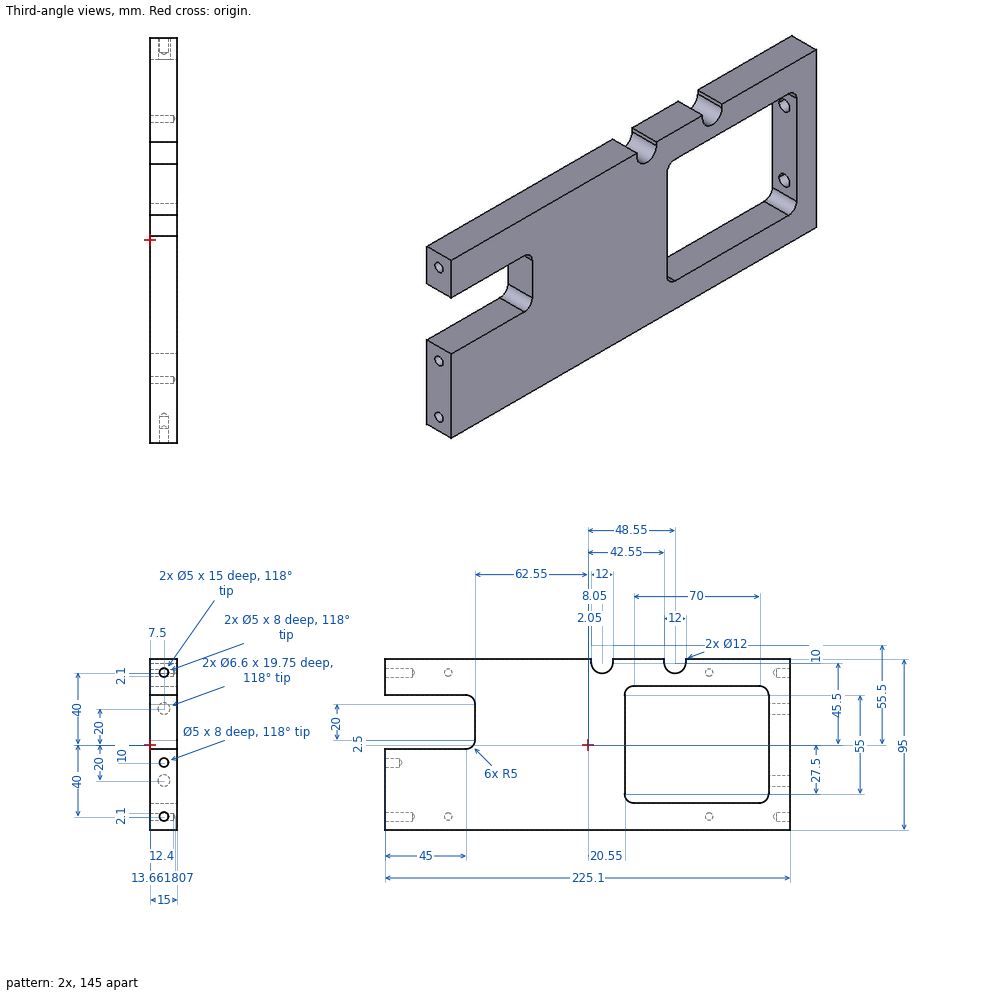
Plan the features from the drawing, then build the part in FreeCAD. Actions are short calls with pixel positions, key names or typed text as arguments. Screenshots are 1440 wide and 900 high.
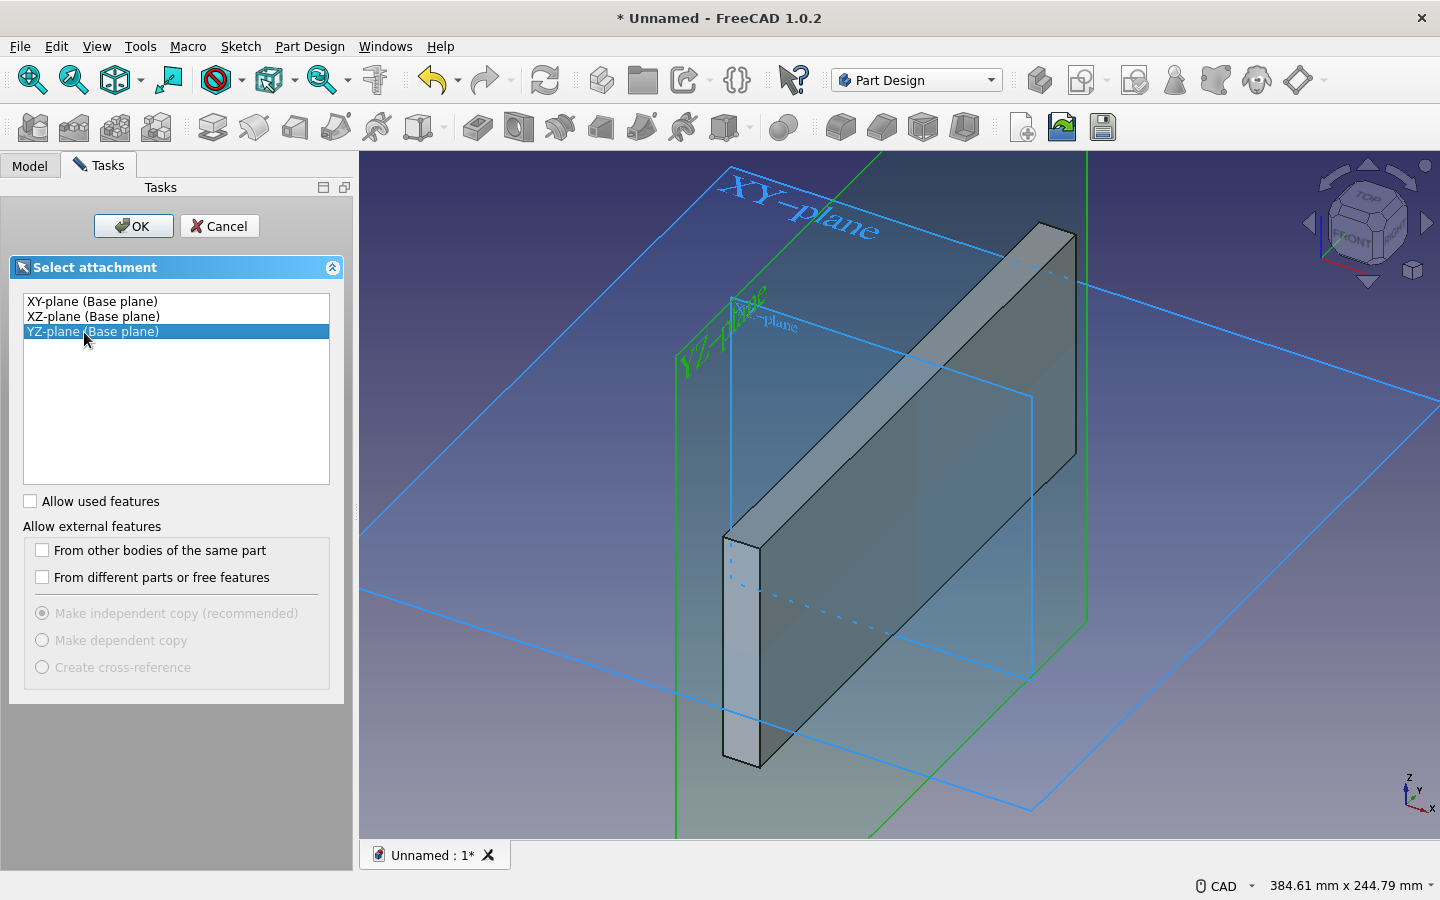
click(134, 226)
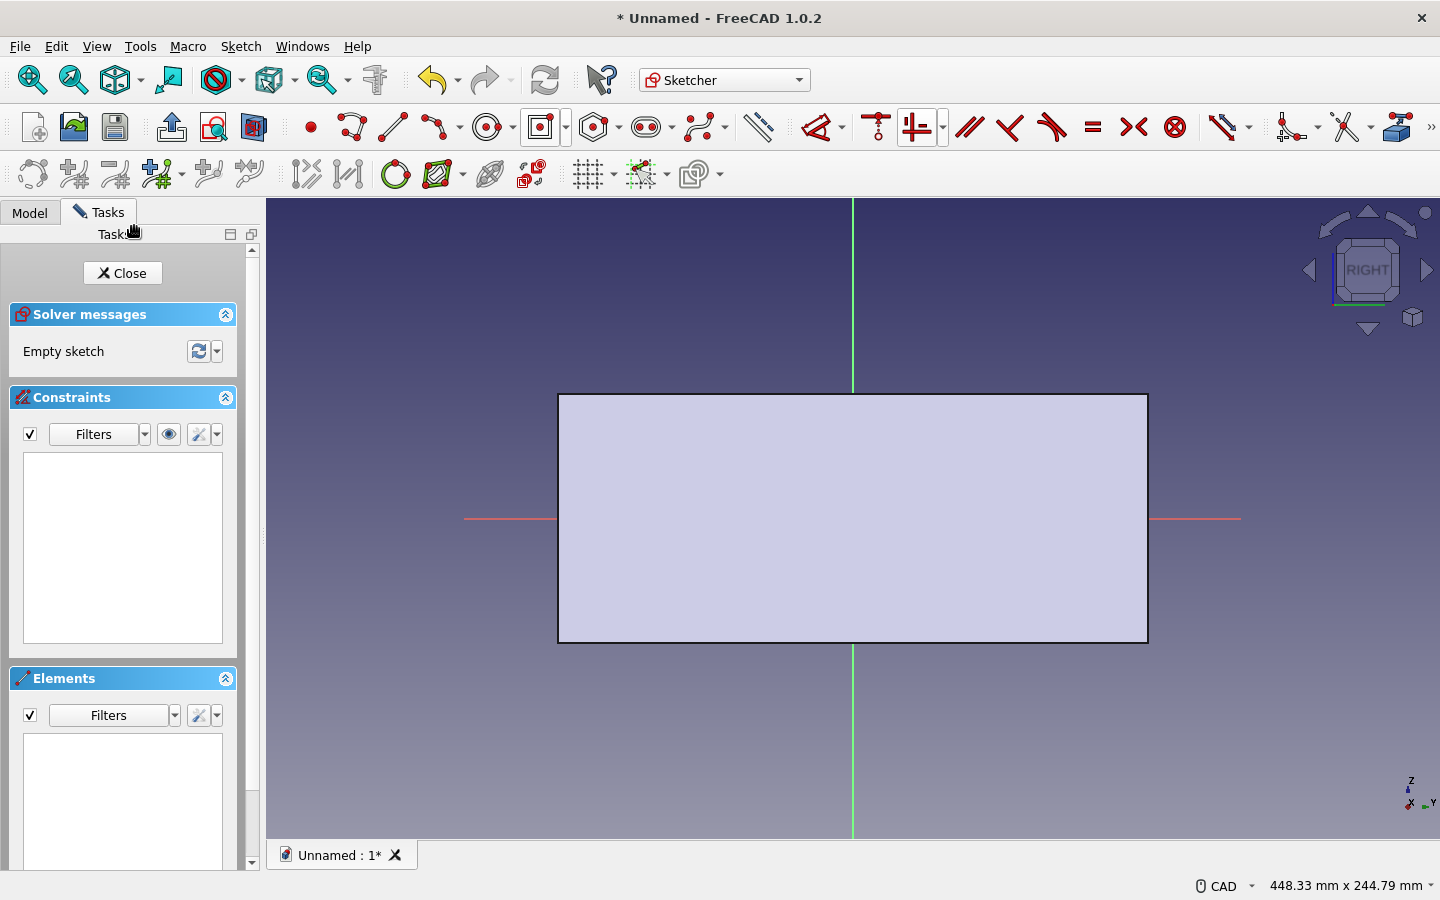
click(254, 128)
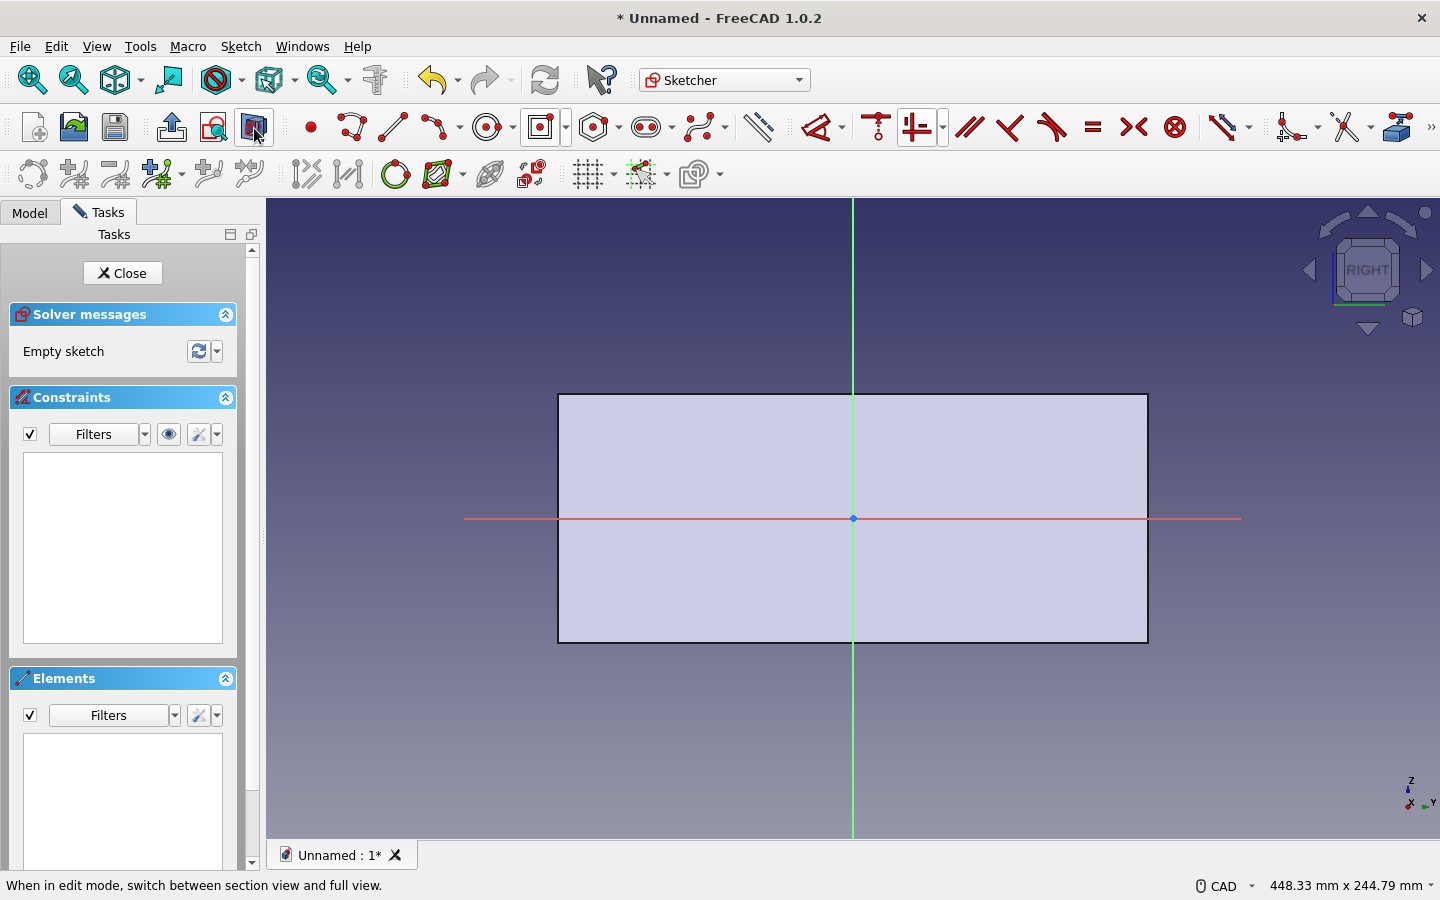
click(393, 128)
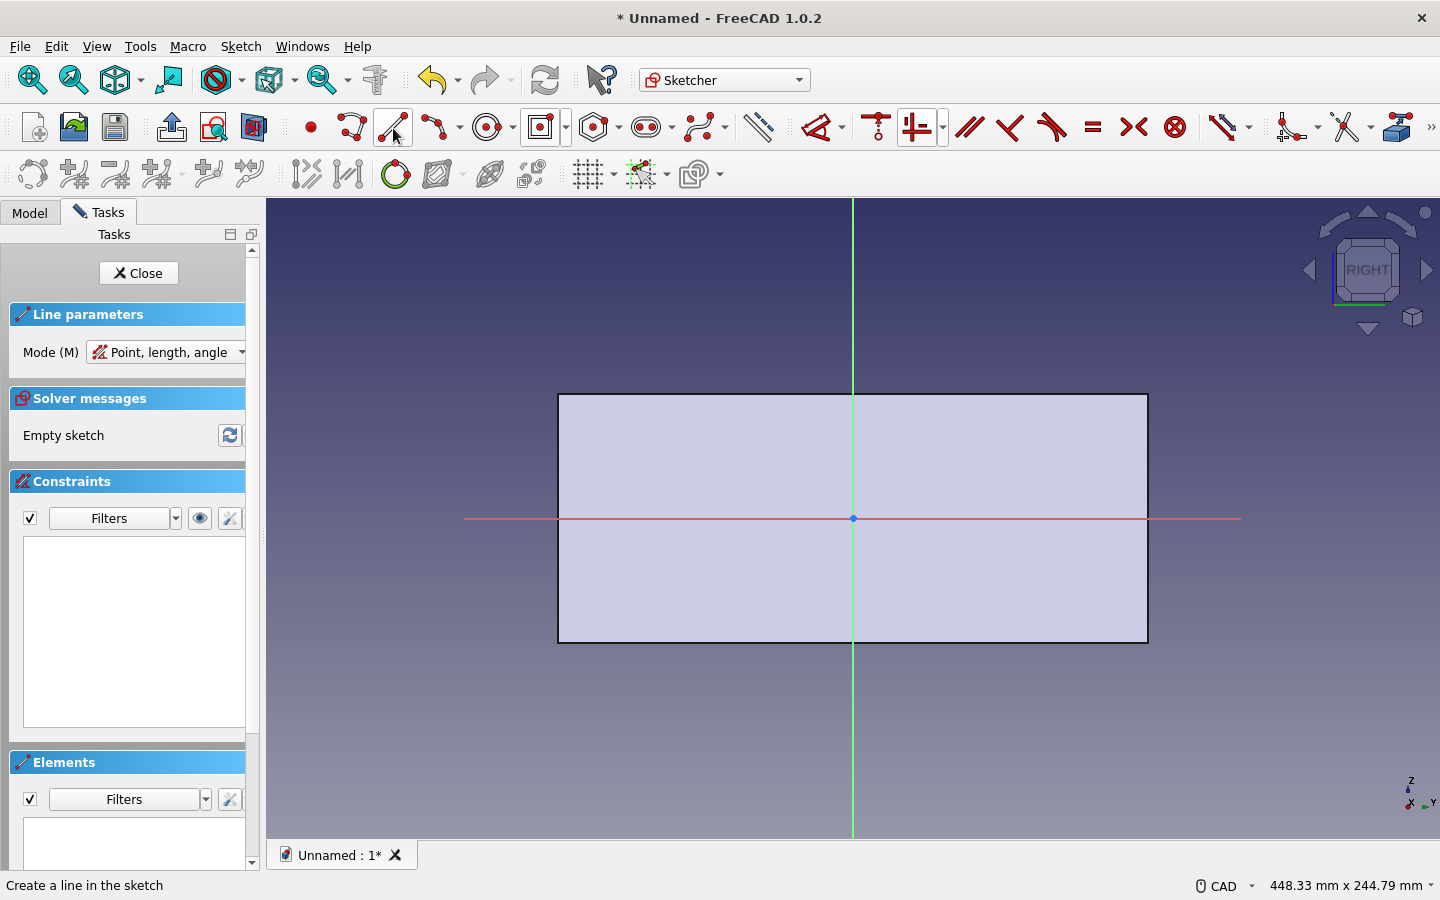
click(689, 460)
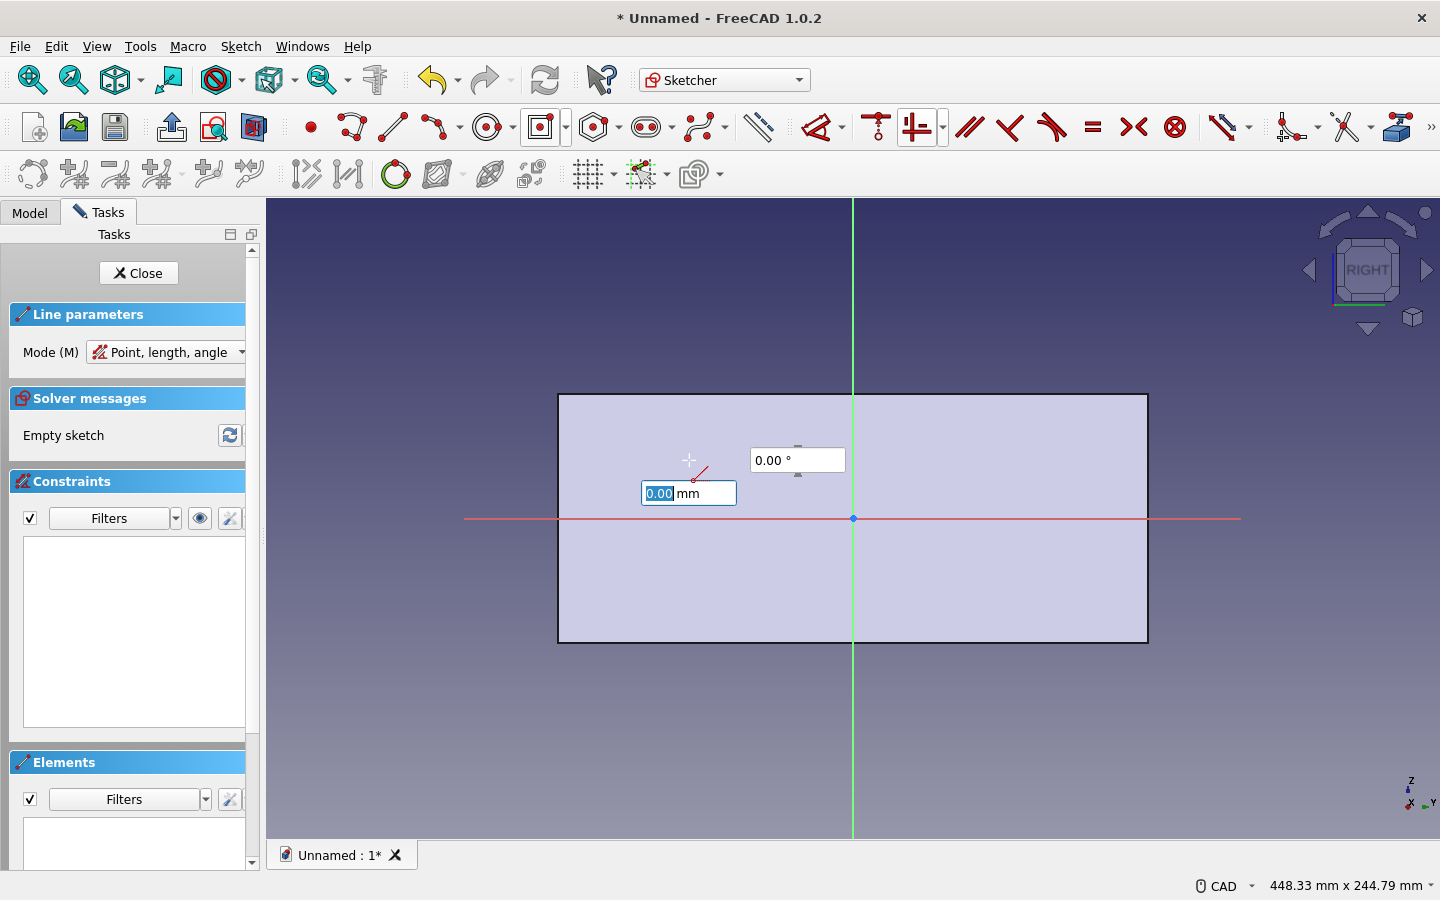
scroll(689, 512, up, 5)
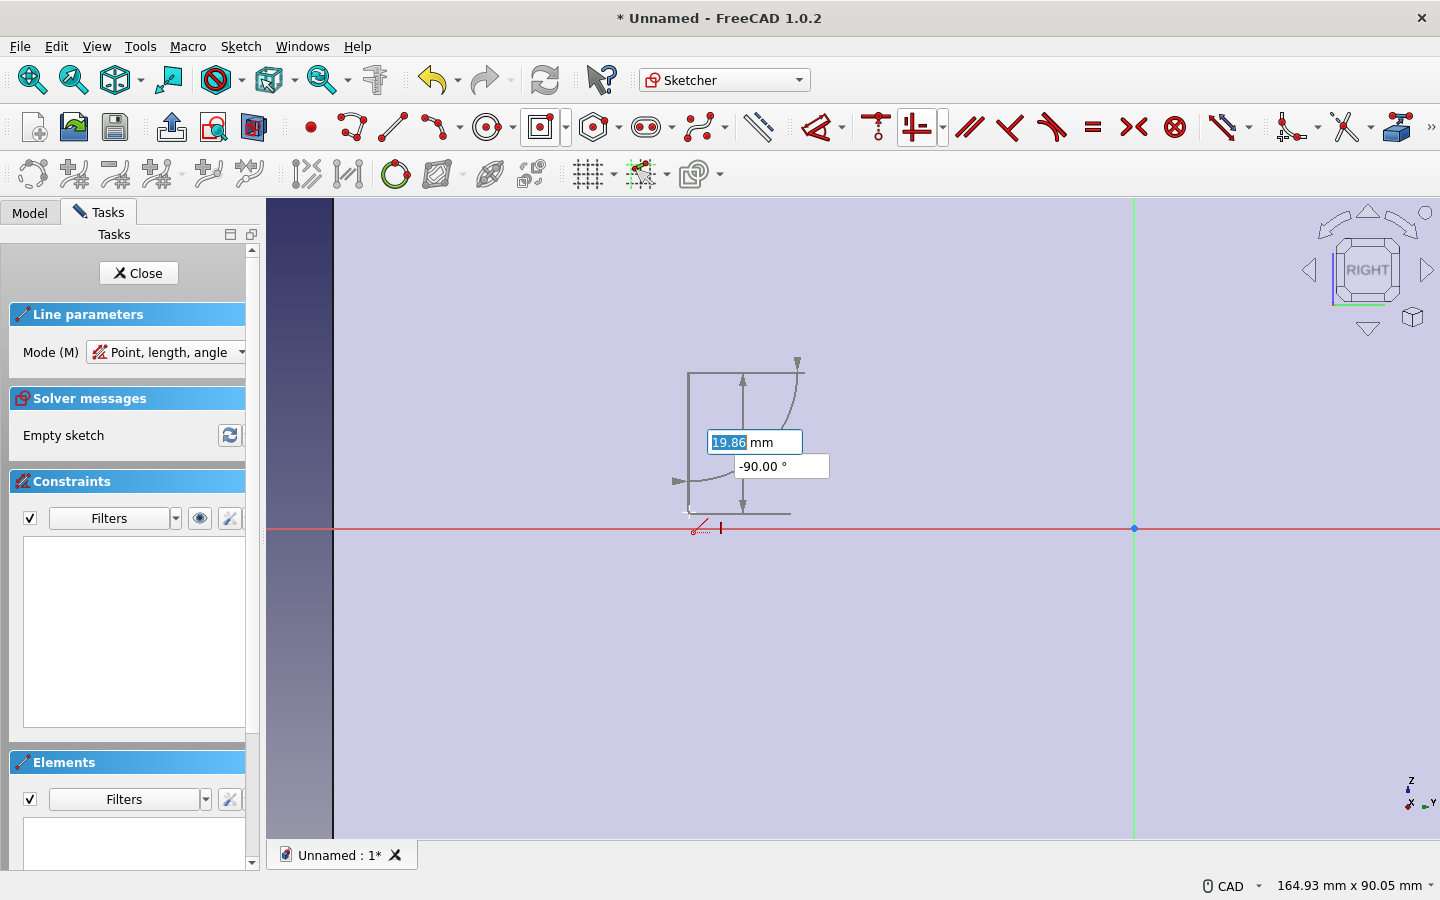
click(688, 511)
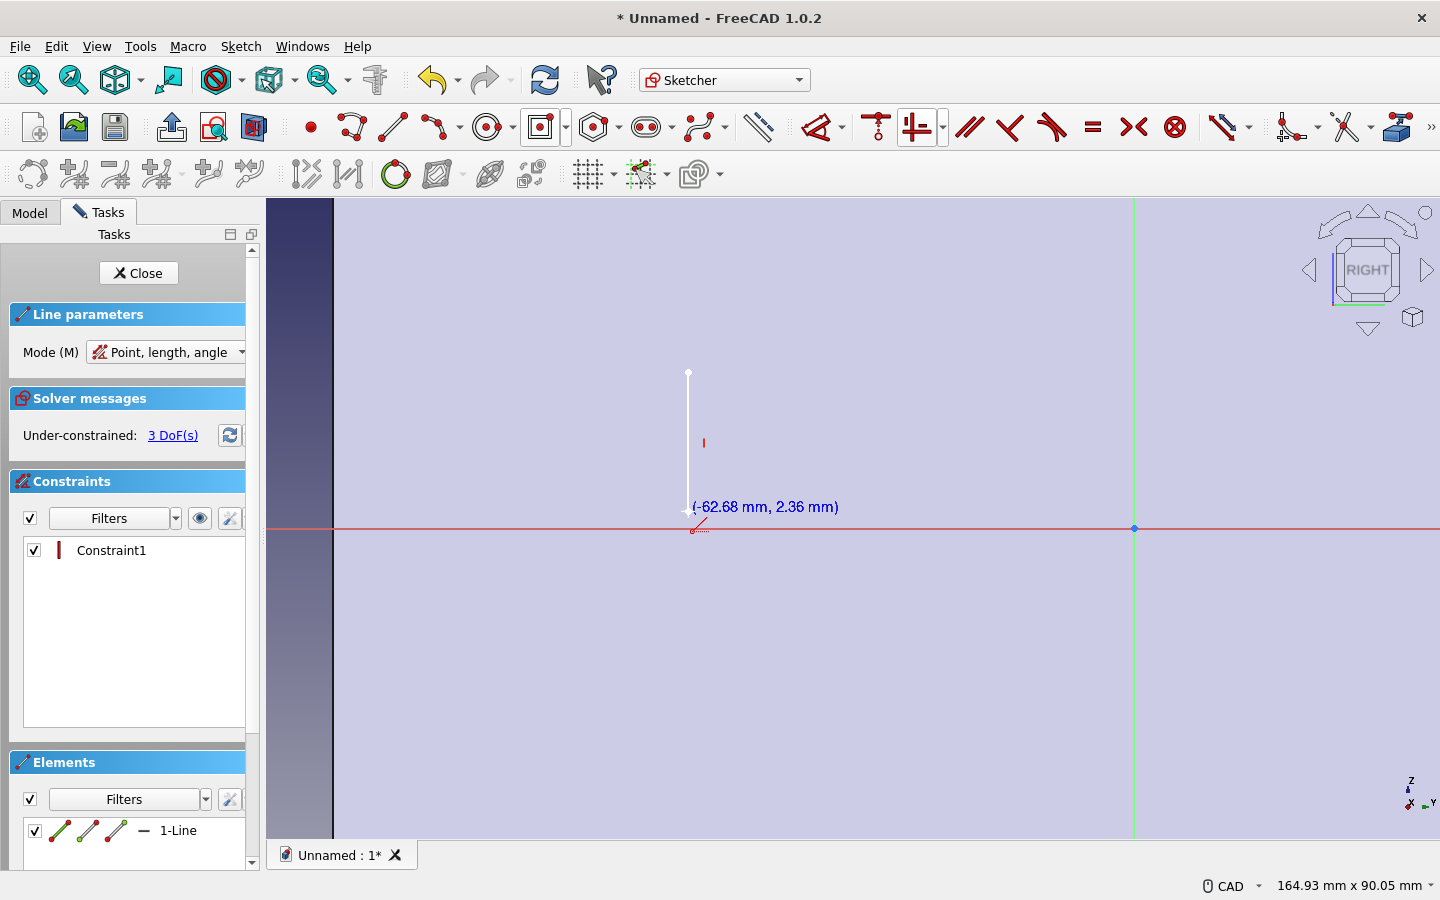
click(352, 128)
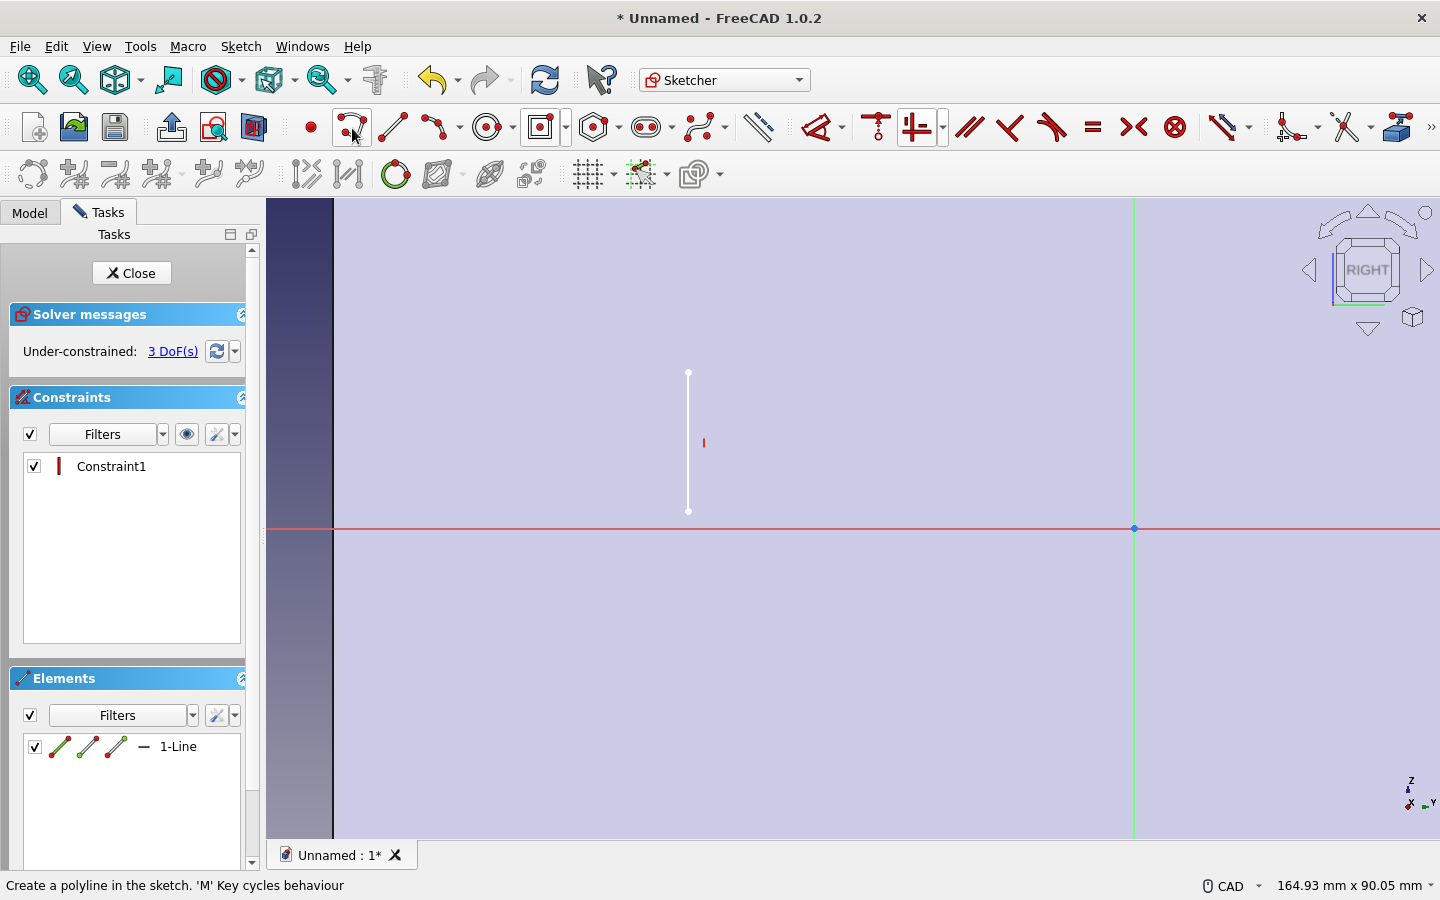
click(653, 547)
click(333, 547)
click(333, 333)
click(653, 333)
right_click(653, 333)